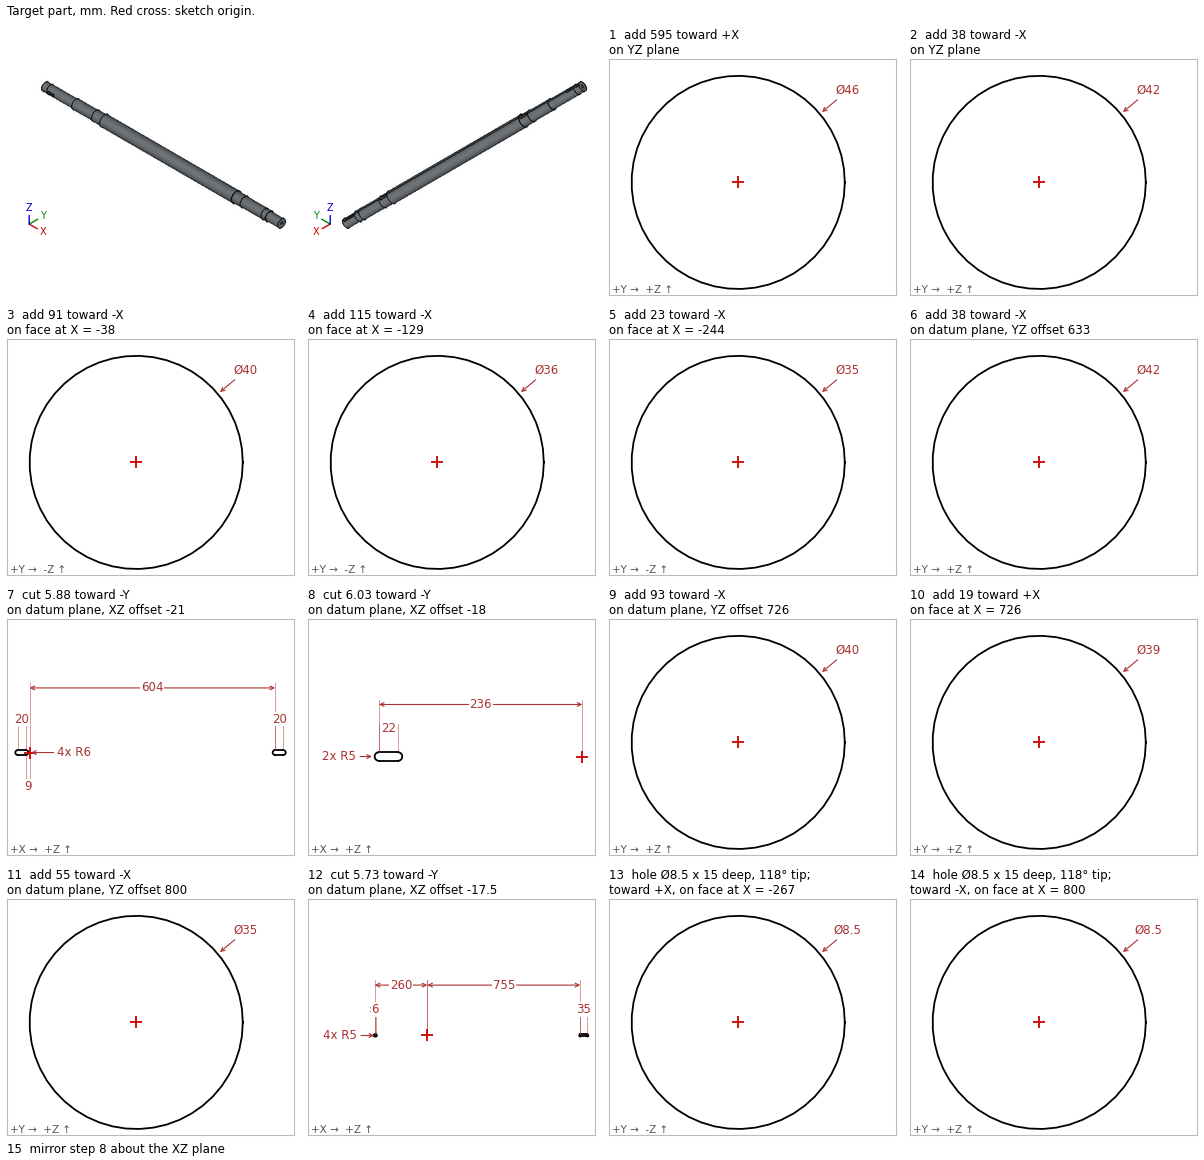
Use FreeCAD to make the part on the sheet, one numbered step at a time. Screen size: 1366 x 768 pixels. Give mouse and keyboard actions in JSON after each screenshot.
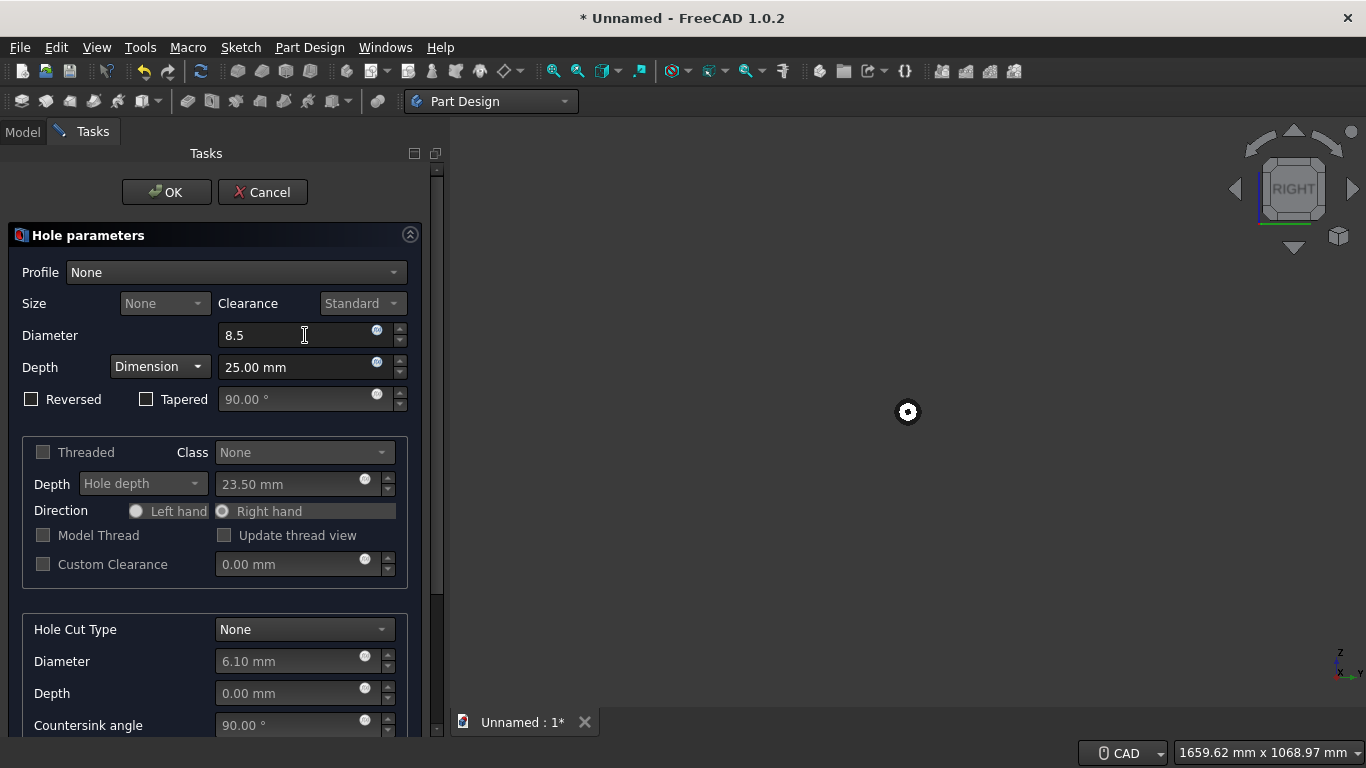
{"action": "triple_click", "coordinate": [305, 367]}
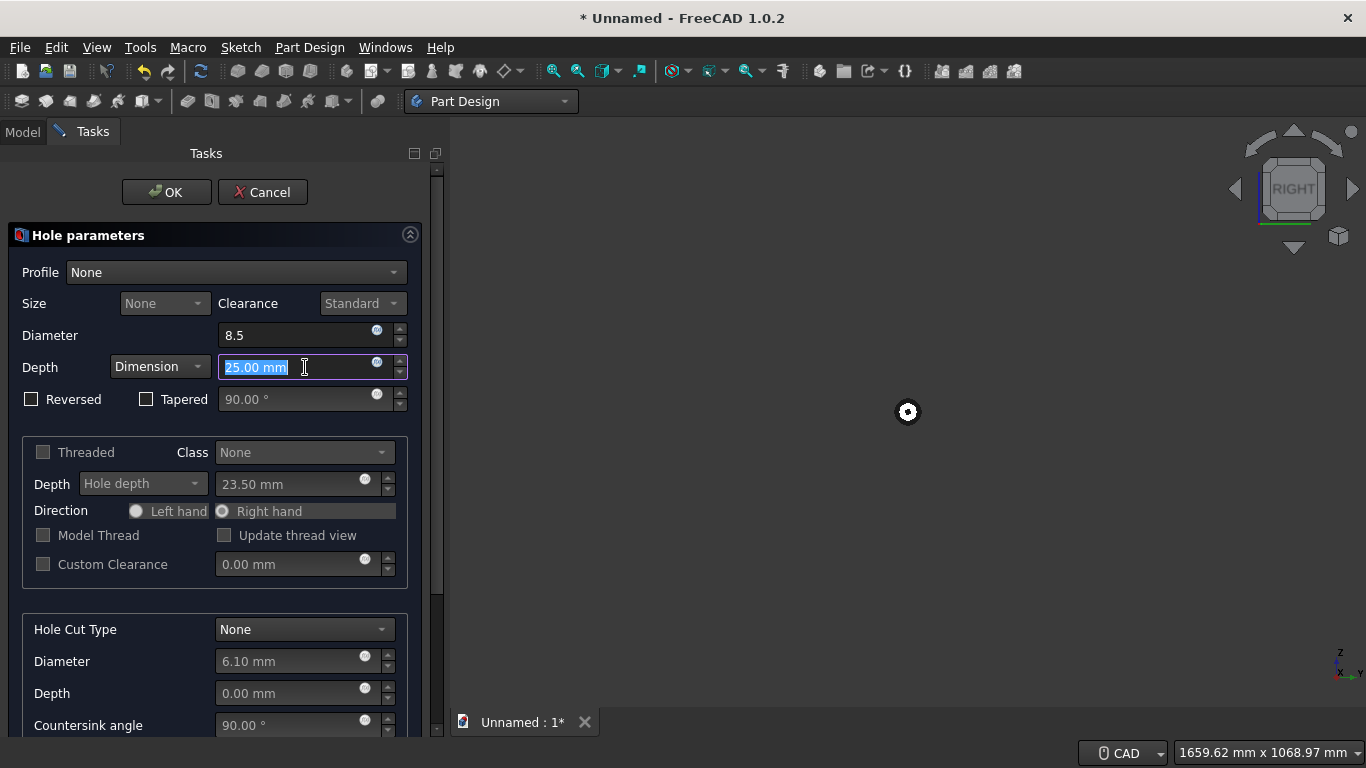
{"action": "type", "text": "15"}
{"action": "key", "text": "Tab"}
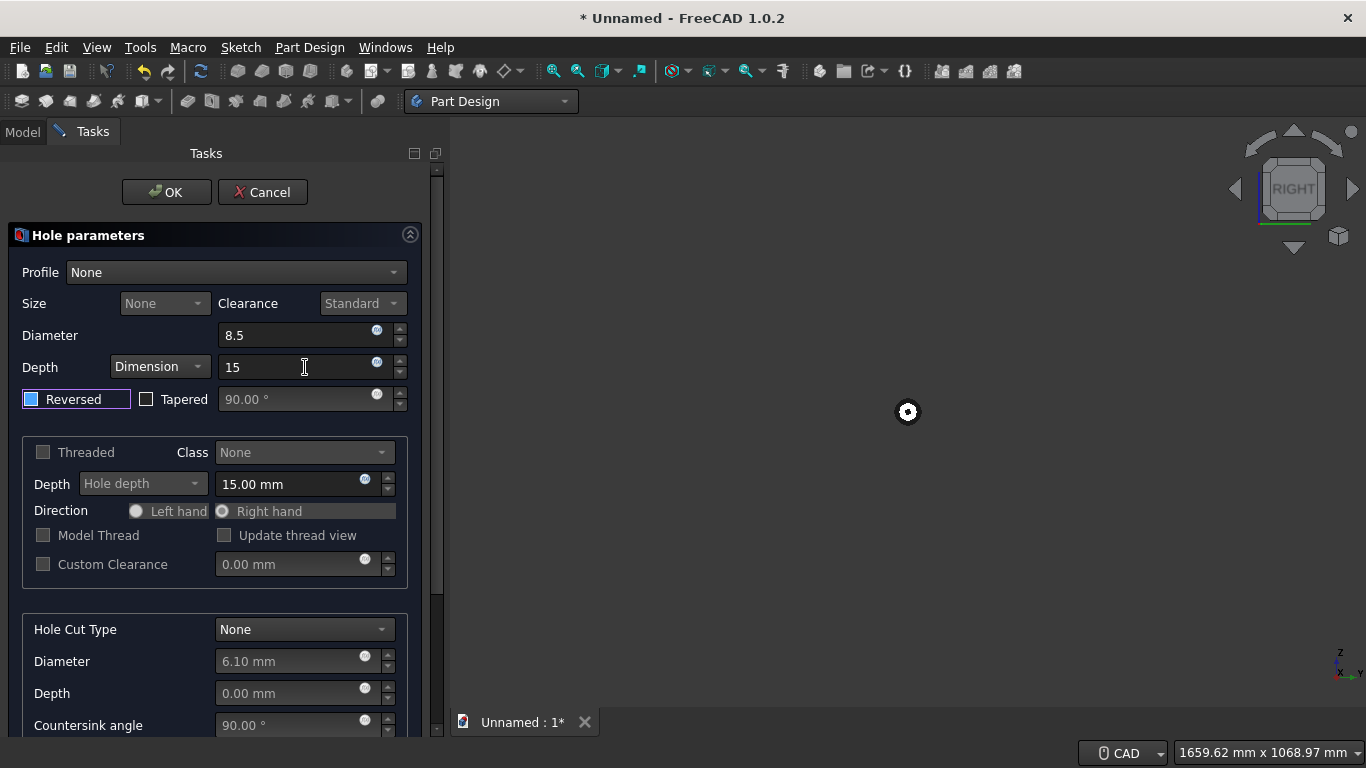
{"action": "left_click", "coordinate": [167, 192]}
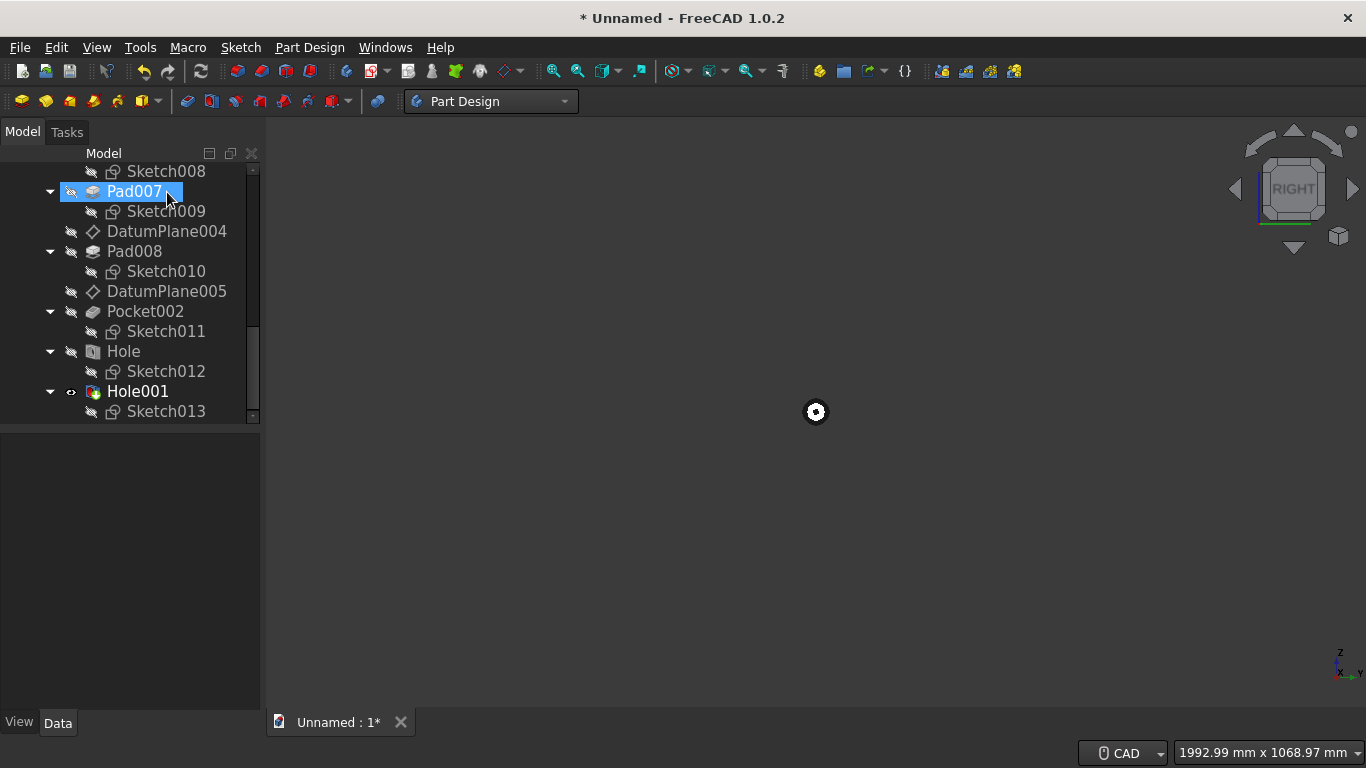
{"action": "left_click", "coordinate": [554, 72]}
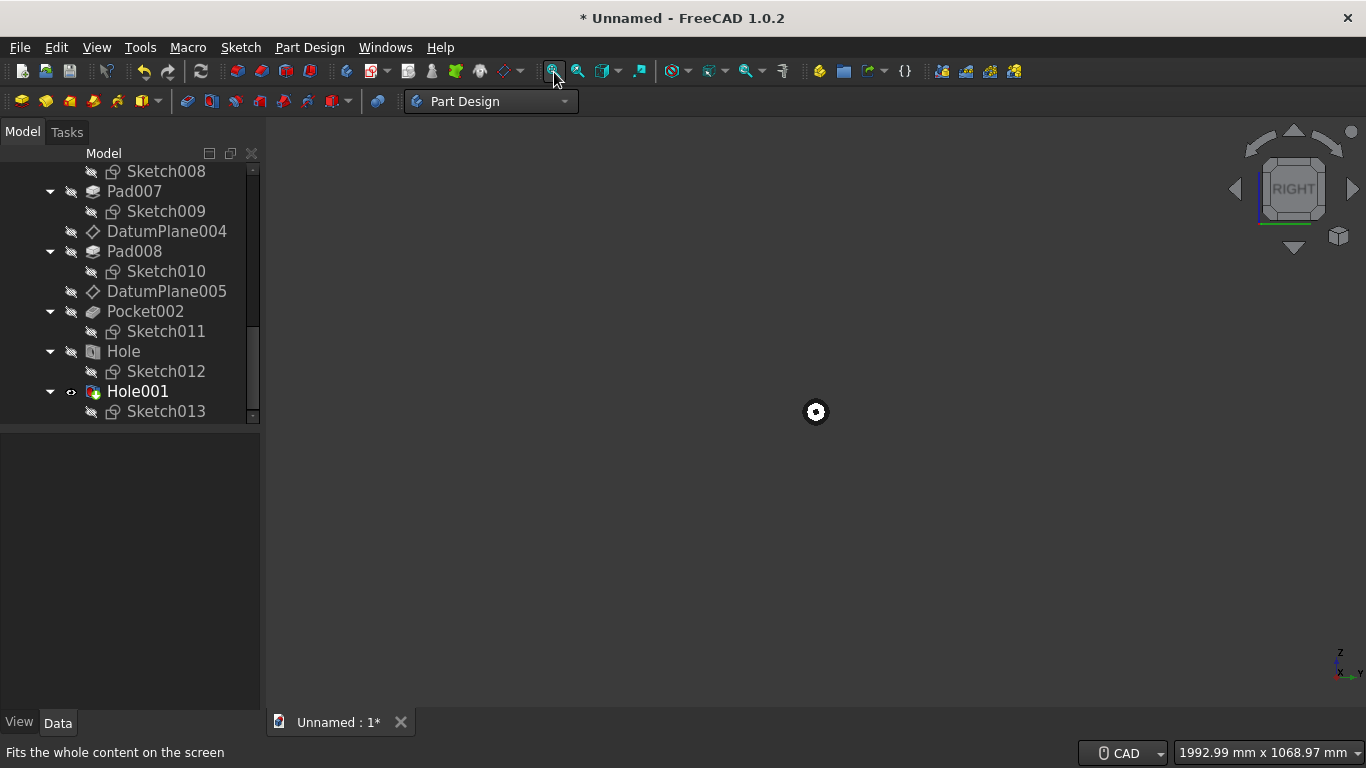
{"action": "scroll", "coordinate": [160, 287], "scroll_direction": "down", "scroll_amount": 3}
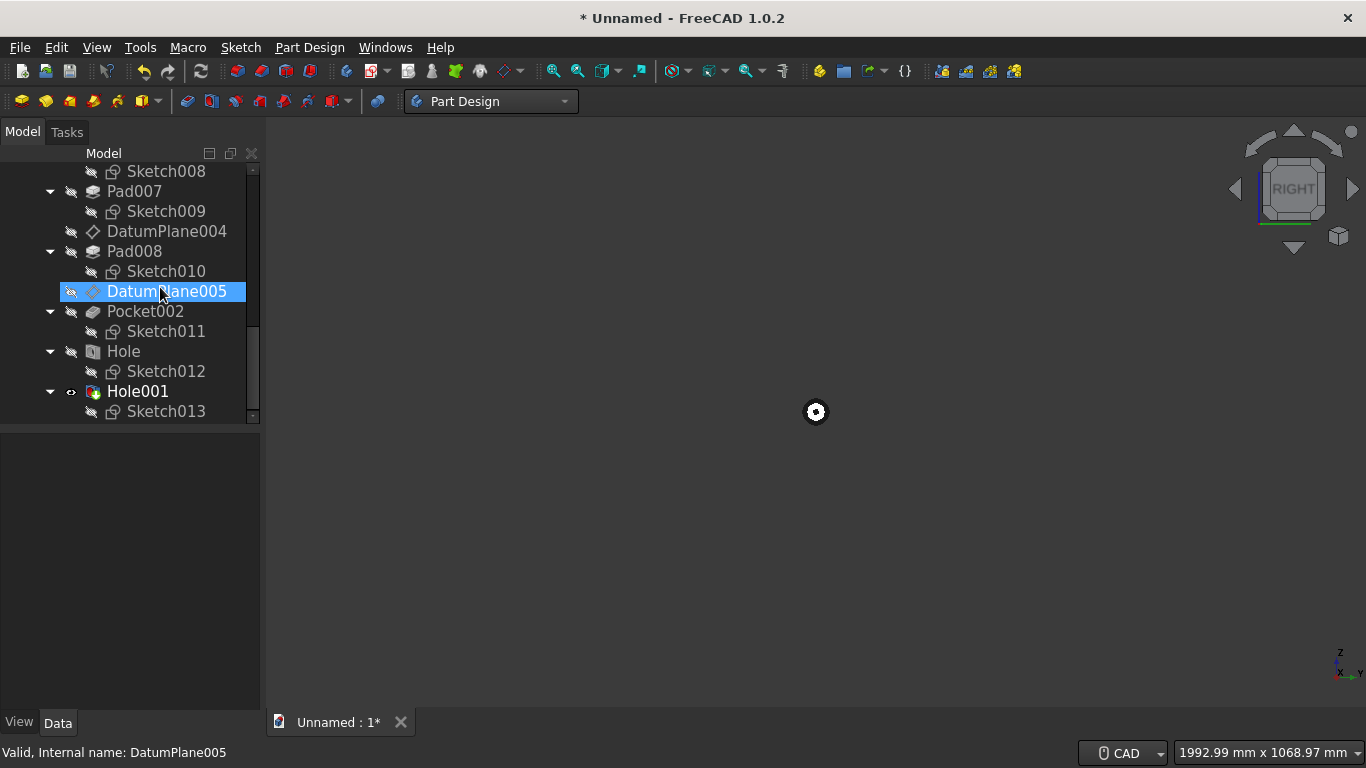
{"action": "scroll", "coordinate": [160, 287], "scroll_direction": "up", "scroll_amount": 15}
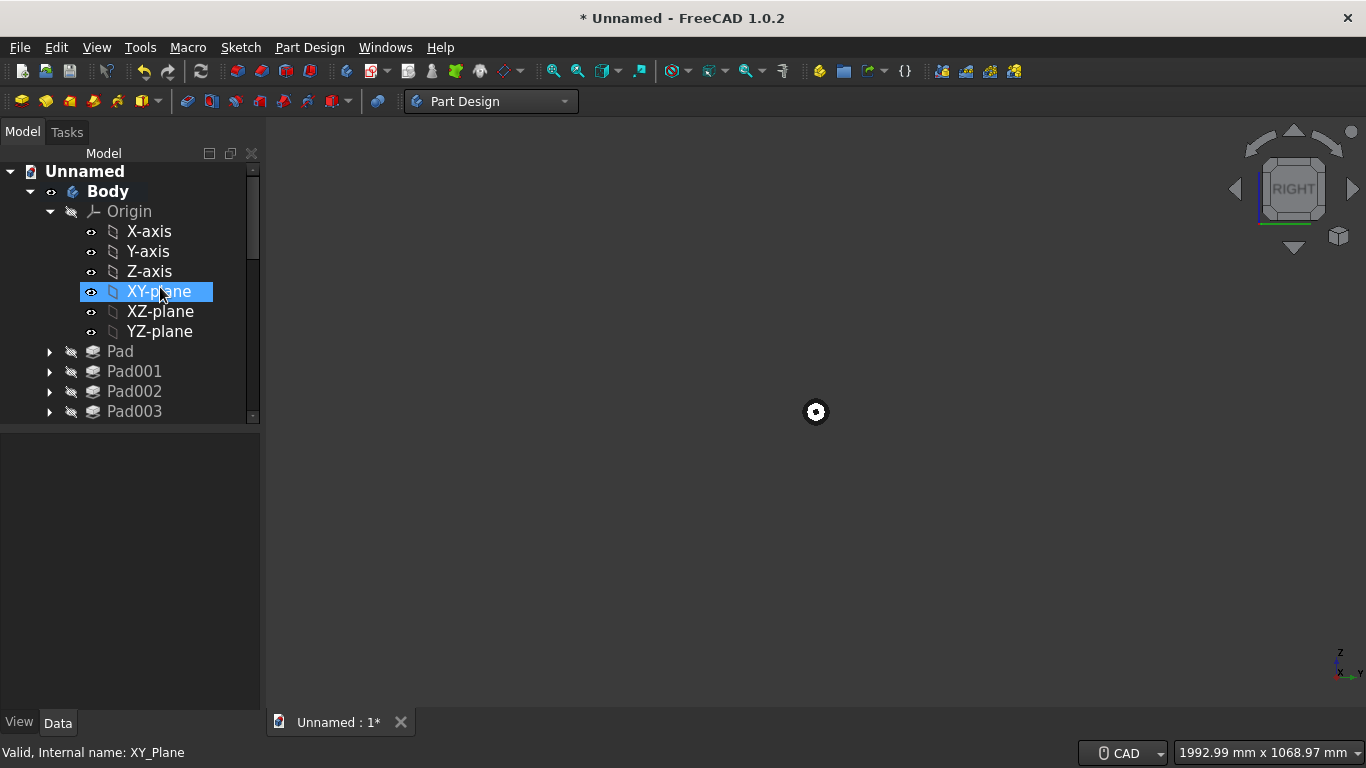
{"action": "scroll", "coordinate": [100, 287], "scroll_direction": "down", "scroll_amount": 6}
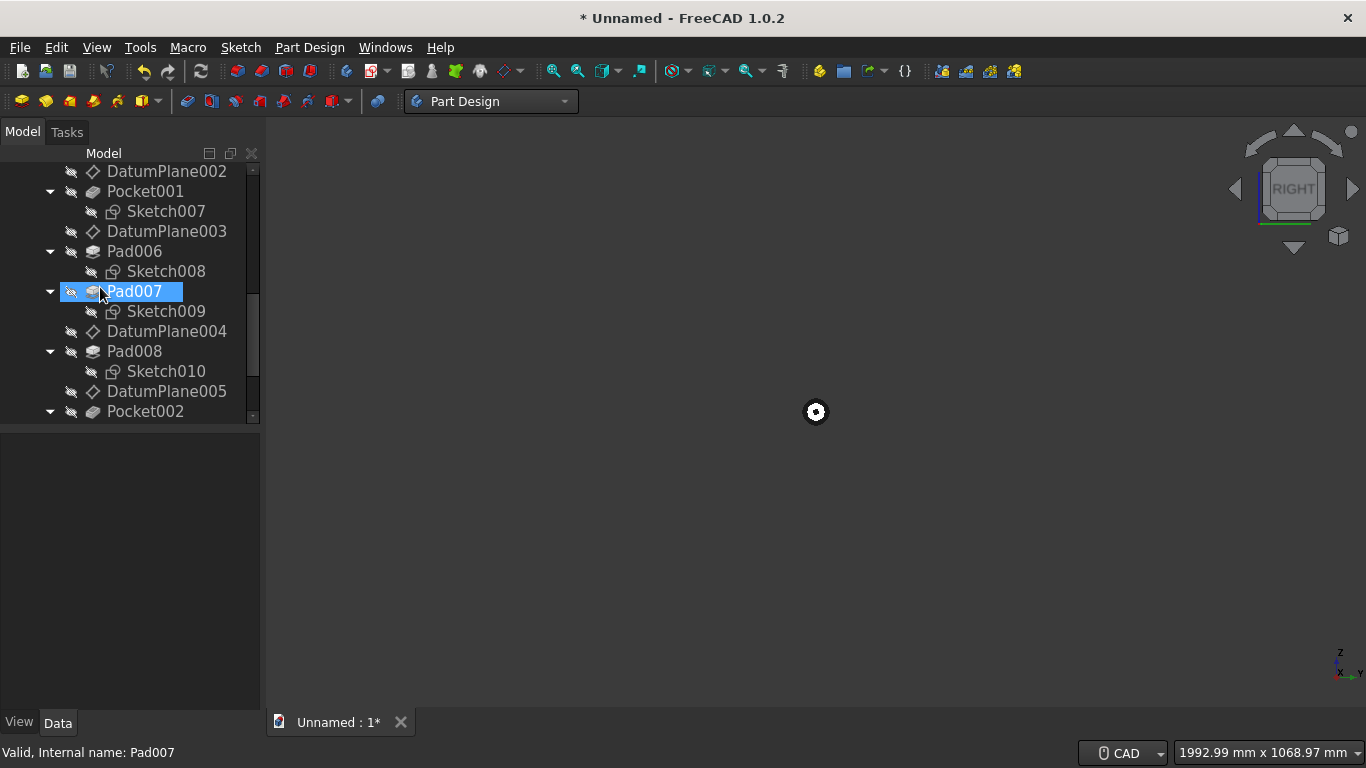
{"action": "left_click", "coordinate": [116, 192]}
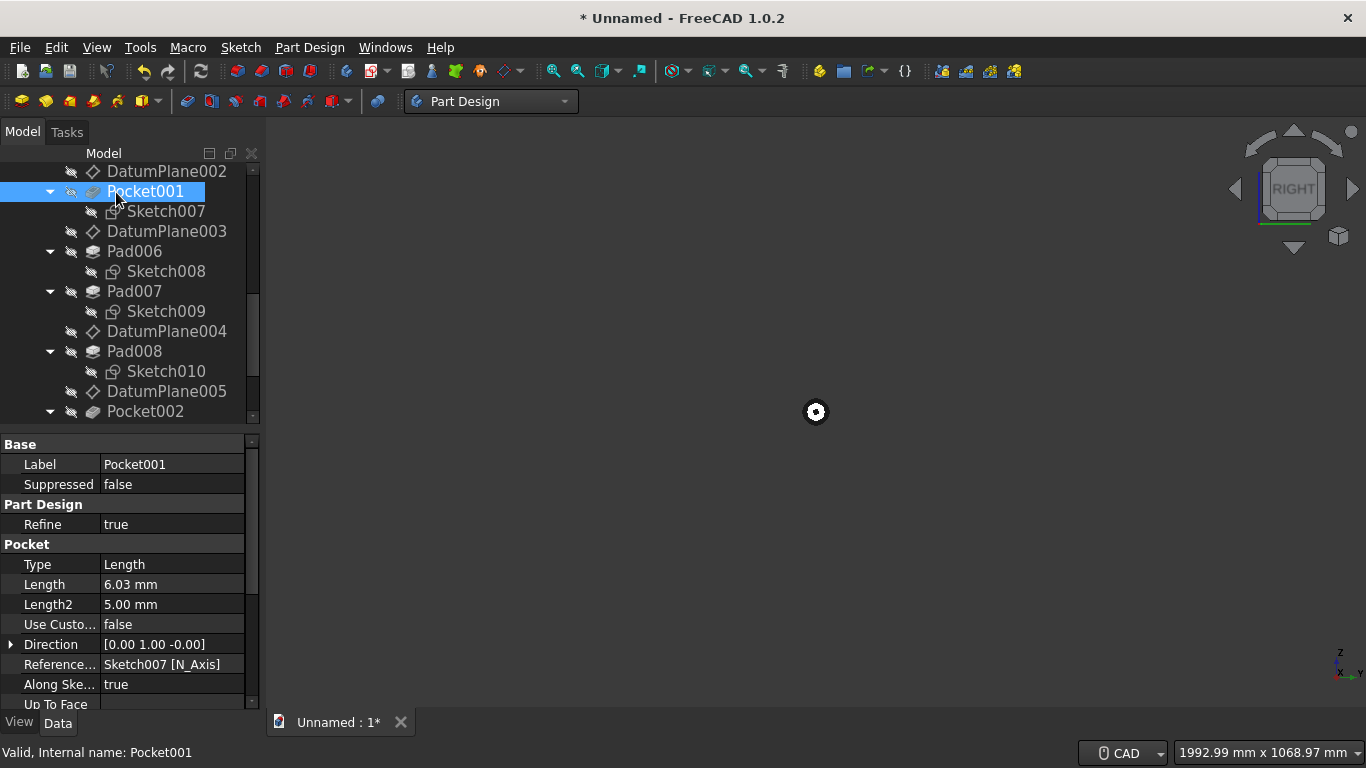
{"action": "left_click", "coordinate": [942, 72]}